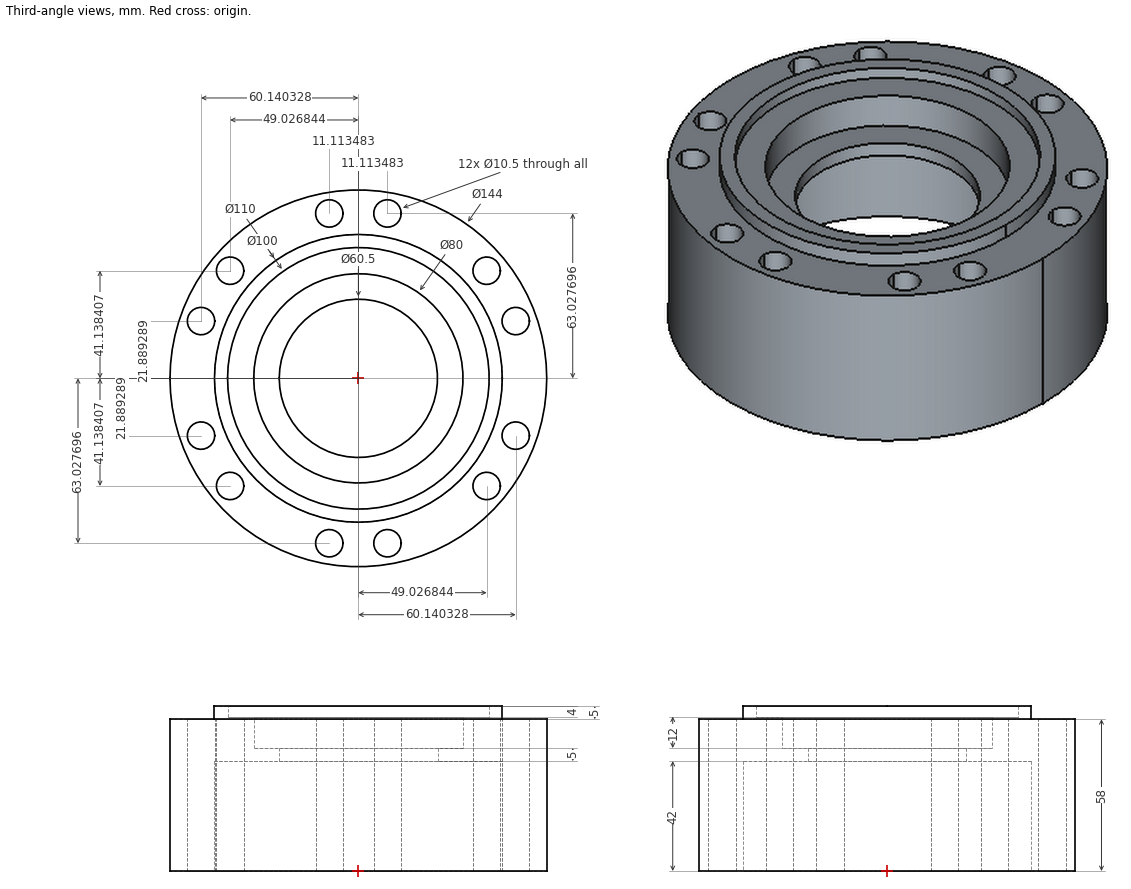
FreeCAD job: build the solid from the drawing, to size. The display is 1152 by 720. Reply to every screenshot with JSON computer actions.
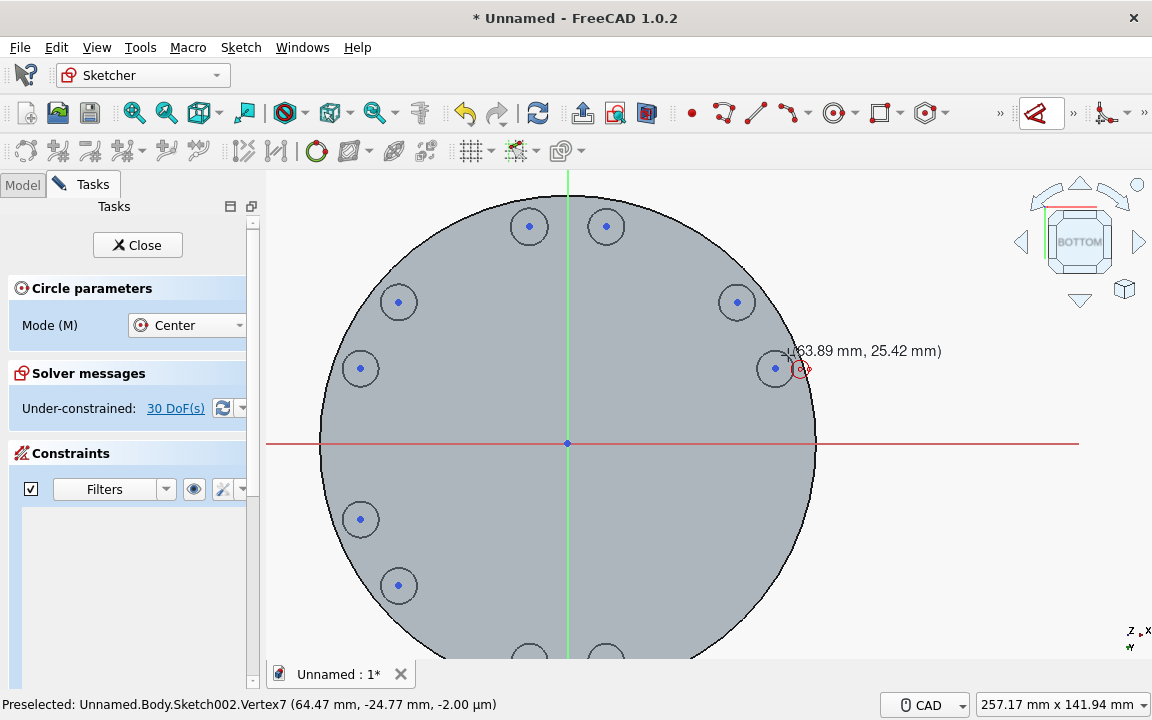
{"action": "scroll", "coordinate": [775, 519], "scroll_direction": "up", "scroll_amount": 2}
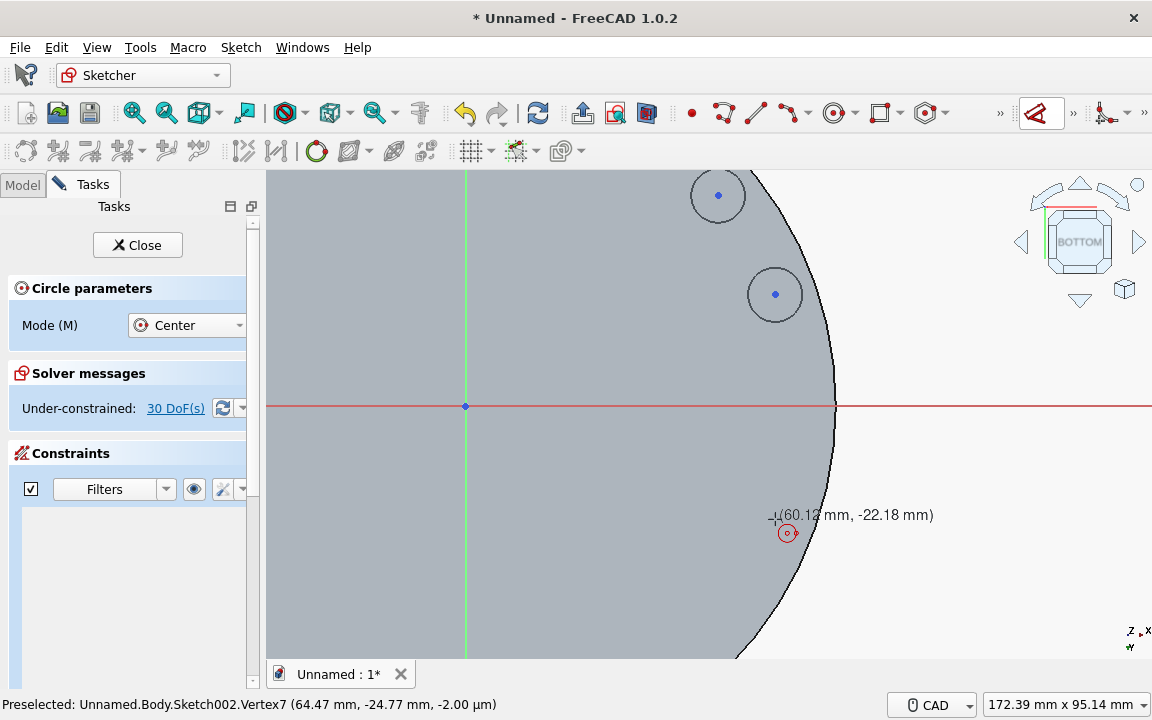
{"action": "left_click", "coordinate": [775, 519]}
{"action": "left_click", "coordinate": [794, 500]}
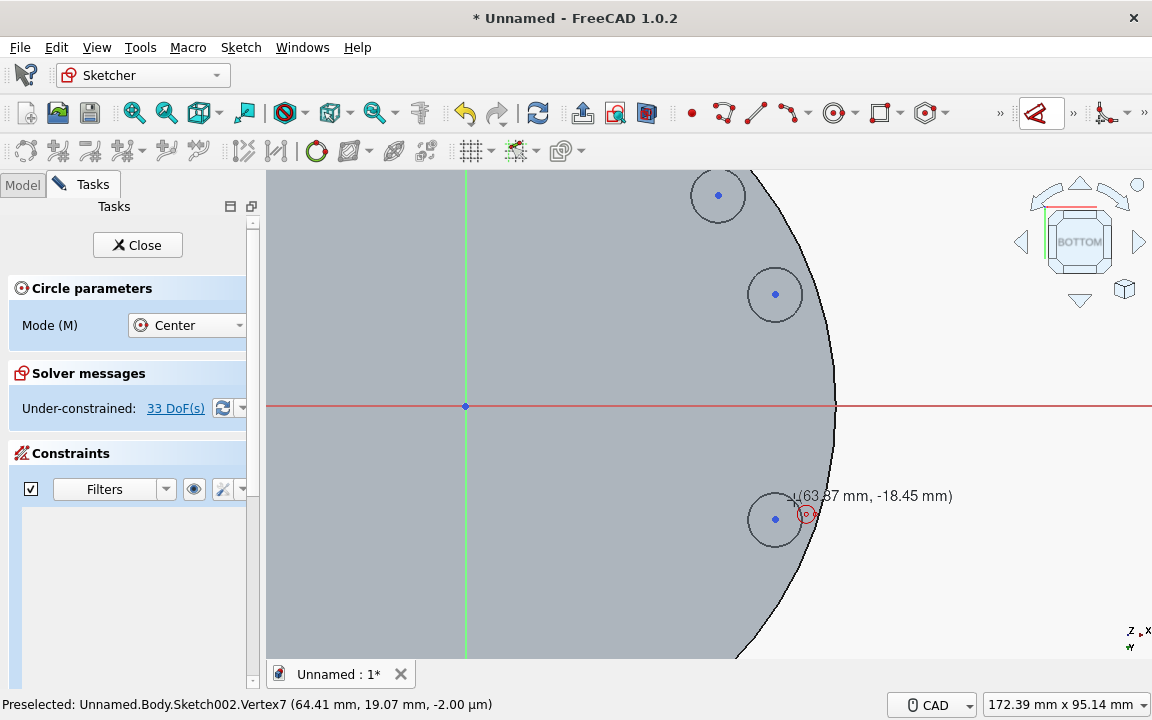
{"action": "left_click", "coordinate": [718, 618]}
{"action": "left_click", "coordinate": [737, 599]}
{"action": "key", "text": "Escape"}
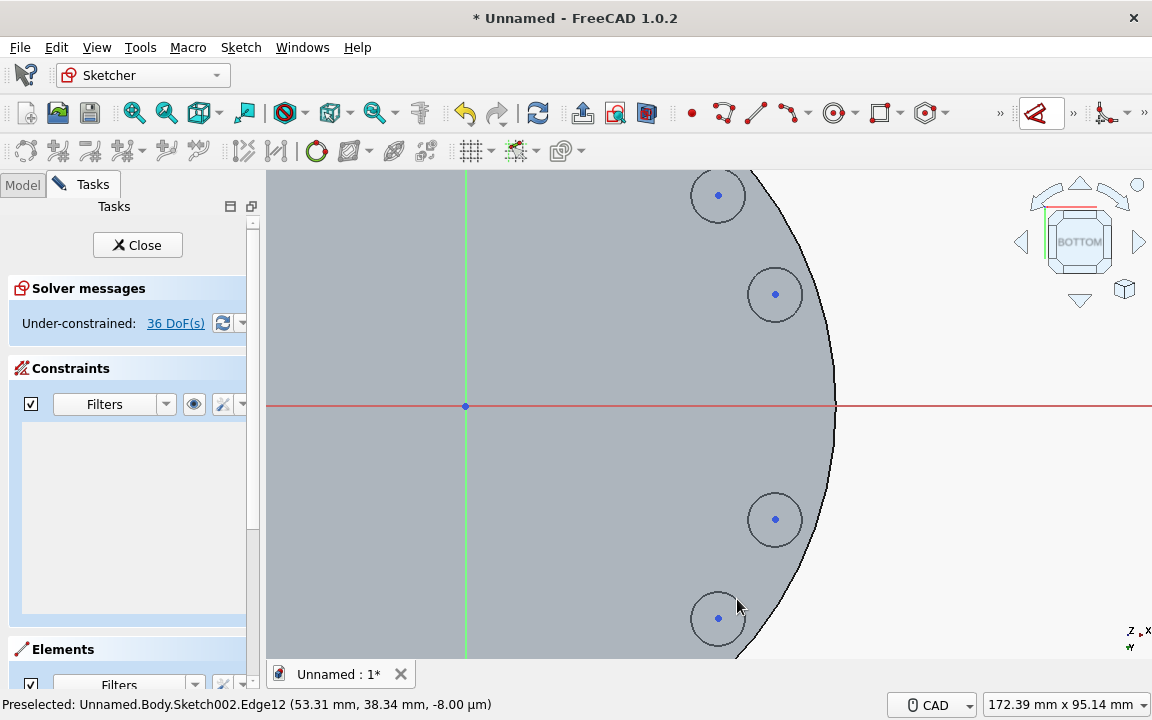
{"action": "scroll", "coordinate": [783, 421], "scroll_direction": "down", "scroll_amount": 4}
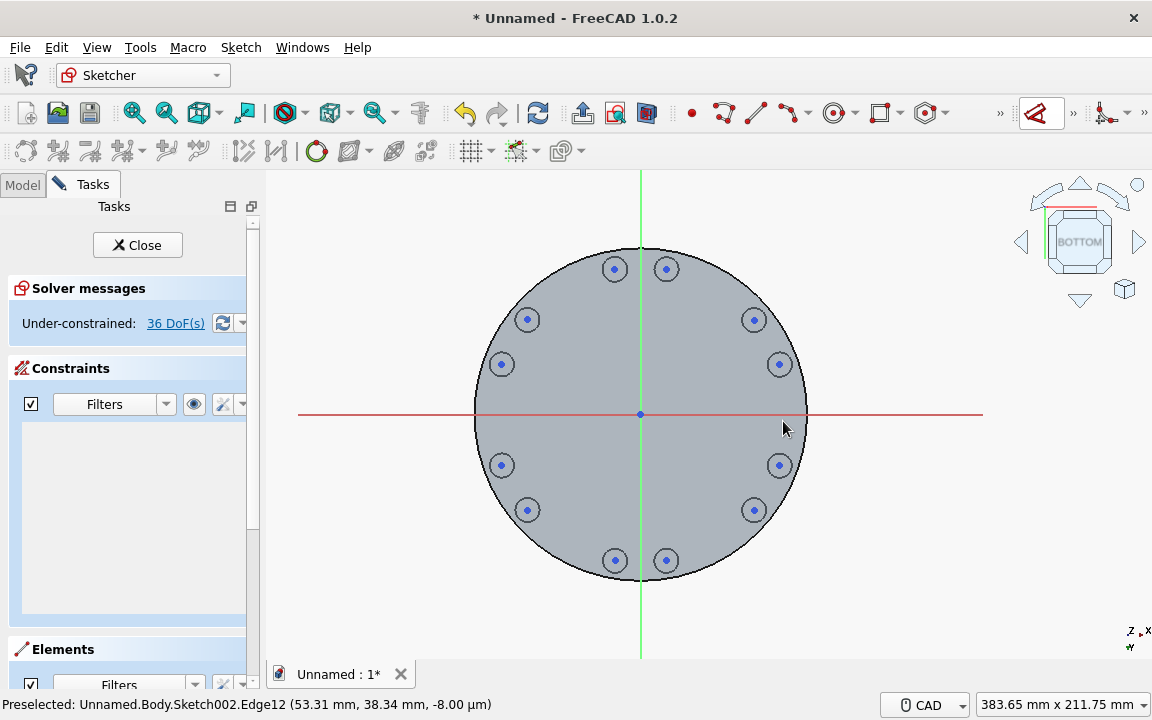
{"action": "left_click", "coordinate": [675, 552]}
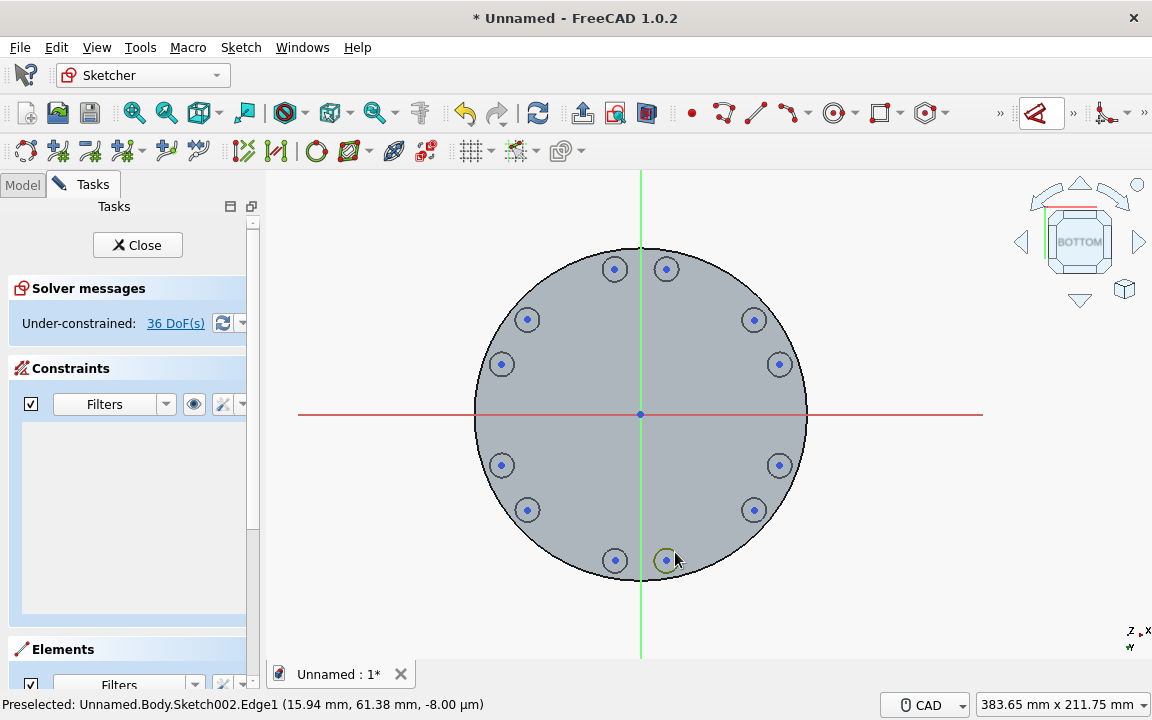
{"action": "left_click", "coordinate": [624, 552]}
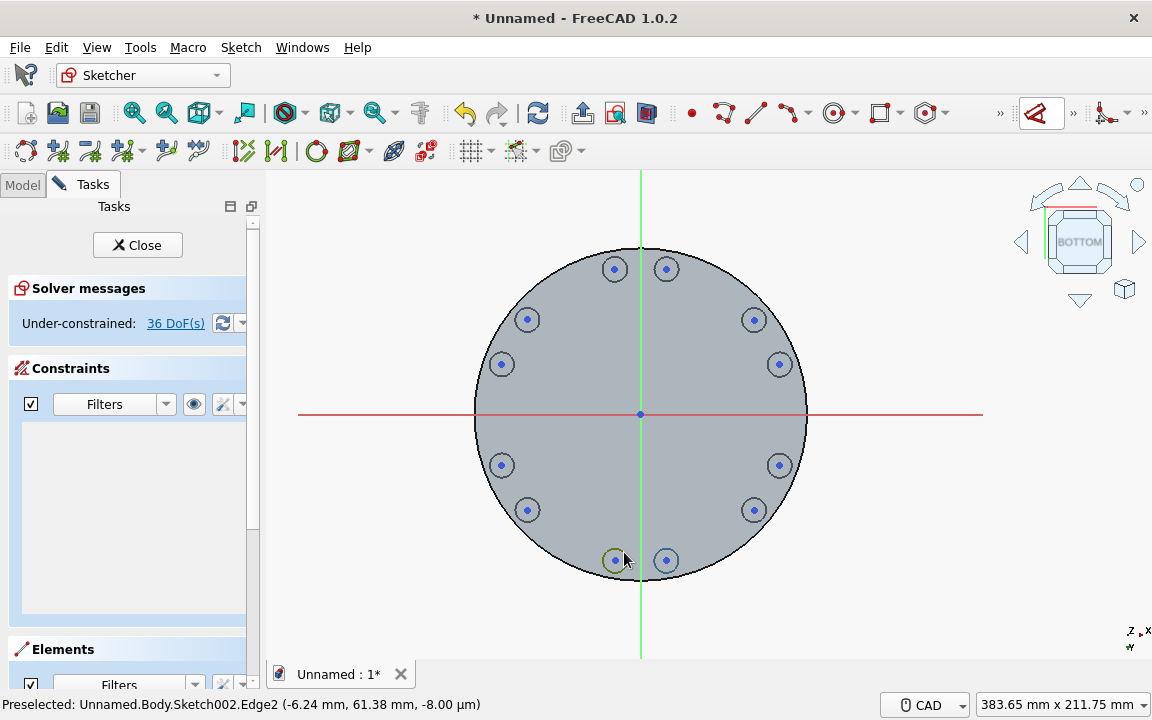
{"action": "left_click", "coordinate": [536, 501]}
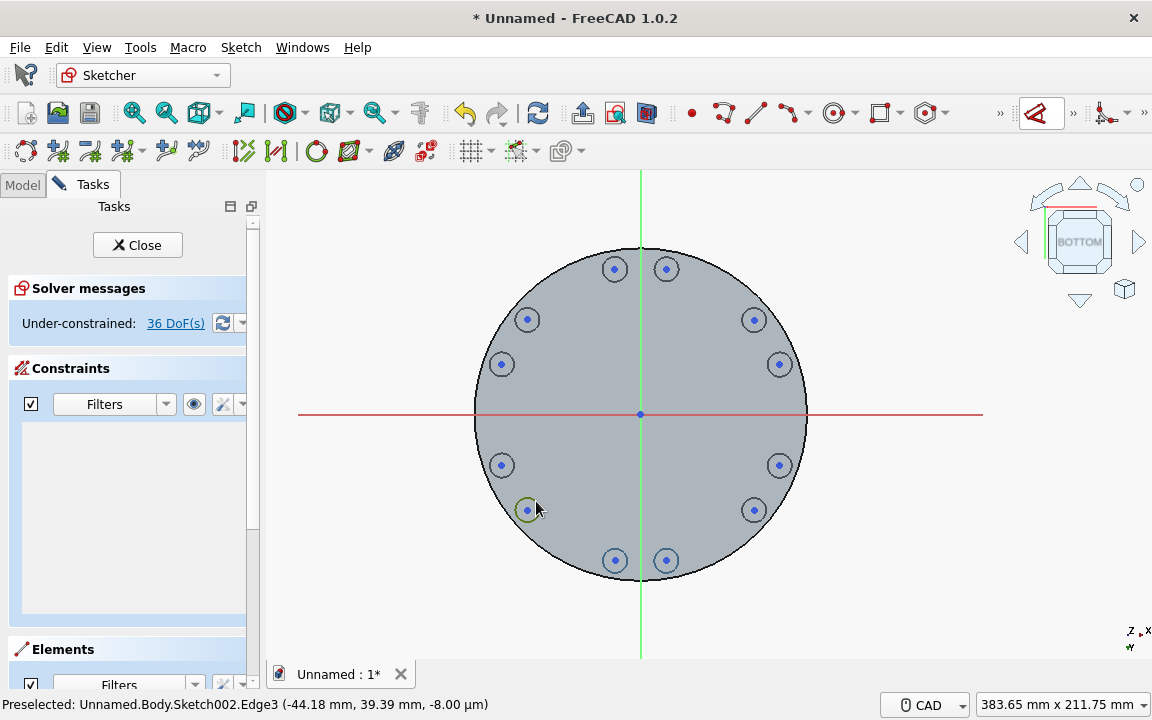
{"action": "left_click", "coordinate": [510, 457]}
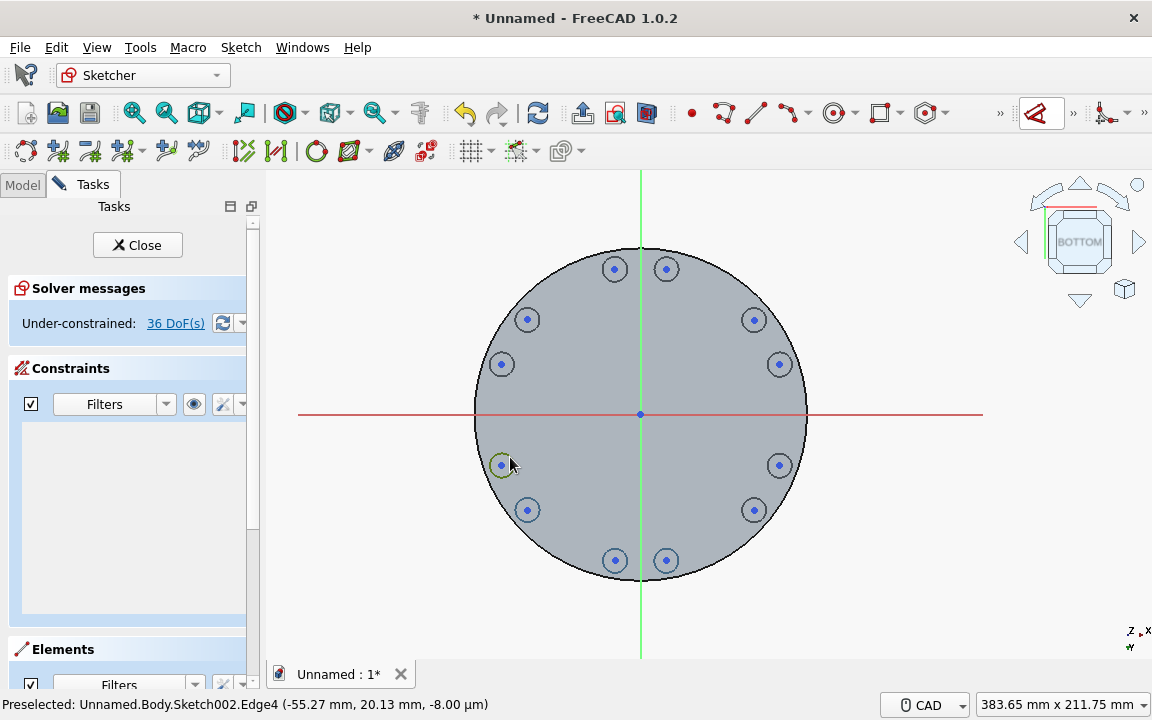
{"action": "left_click", "coordinate": [510, 356]}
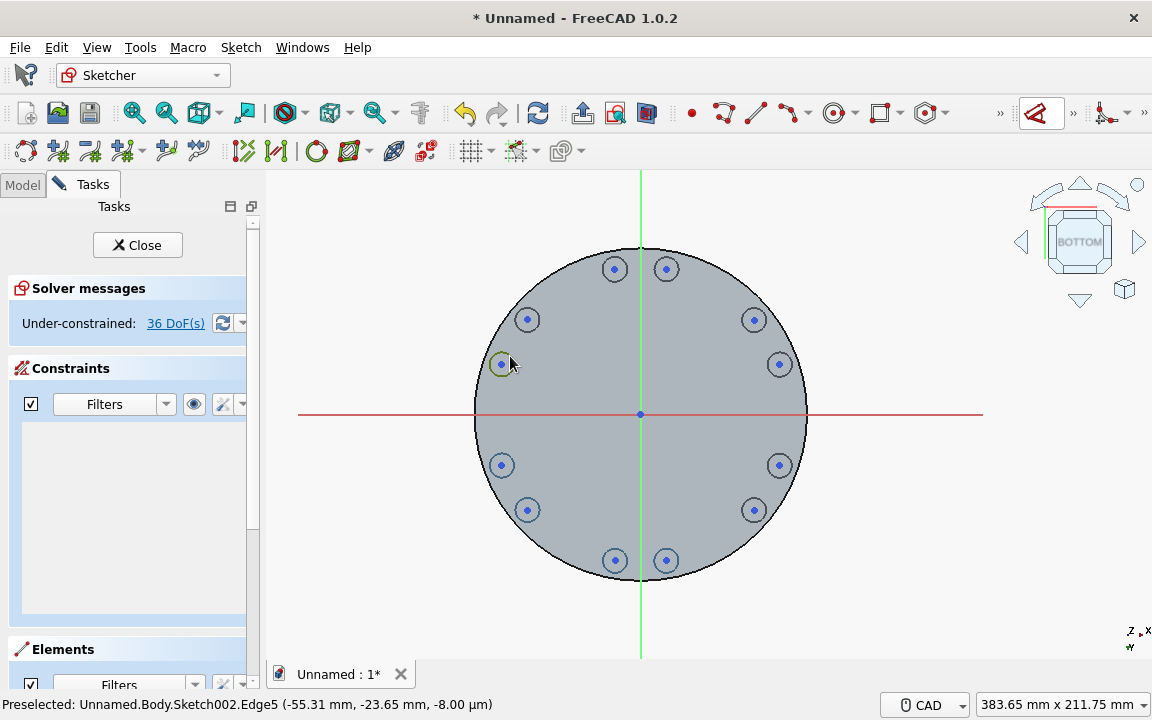
{"action": "left_click", "coordinate": [536, 311]}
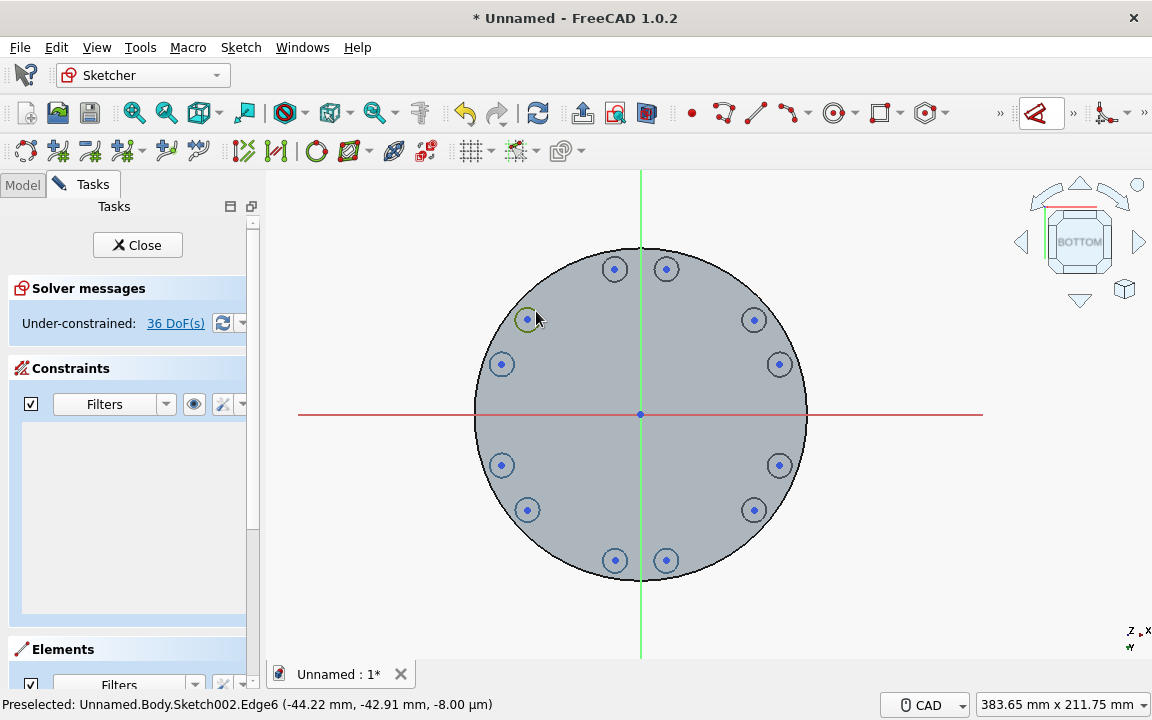
{"action": "left_click", "coordinate": [624, 261]}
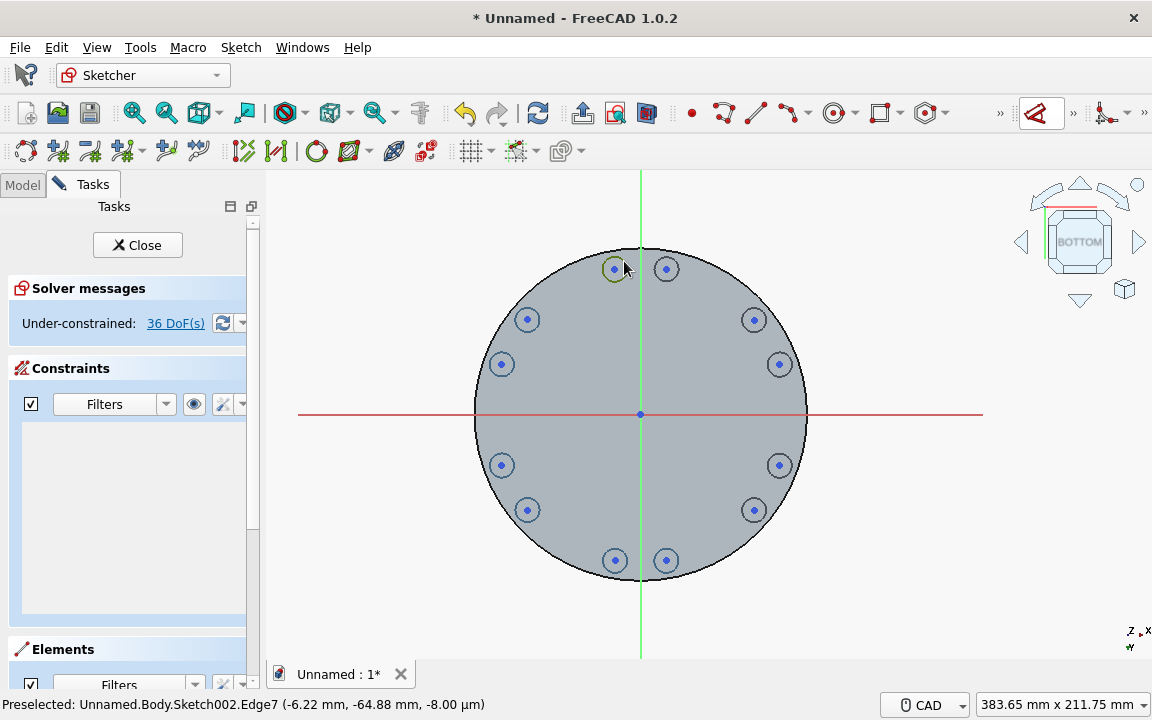
{"action": "left_click", "coordinate": [675, 261]}